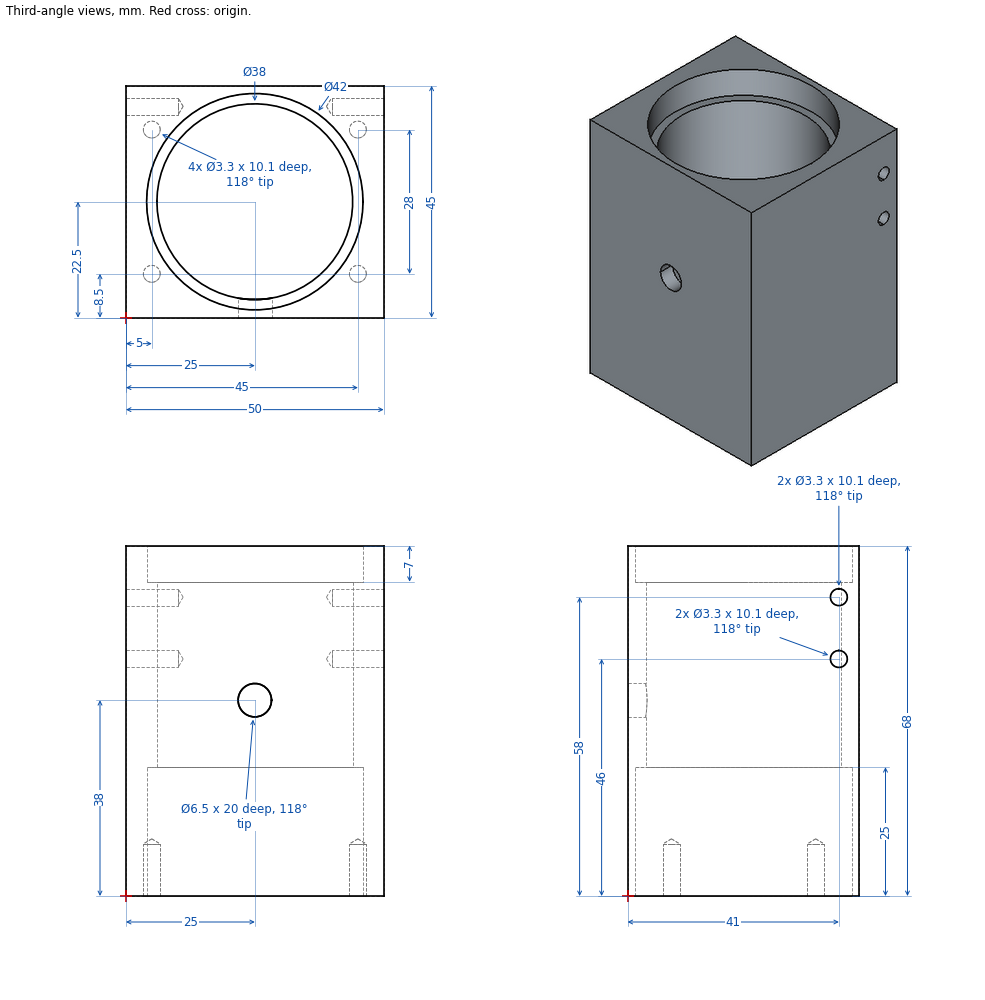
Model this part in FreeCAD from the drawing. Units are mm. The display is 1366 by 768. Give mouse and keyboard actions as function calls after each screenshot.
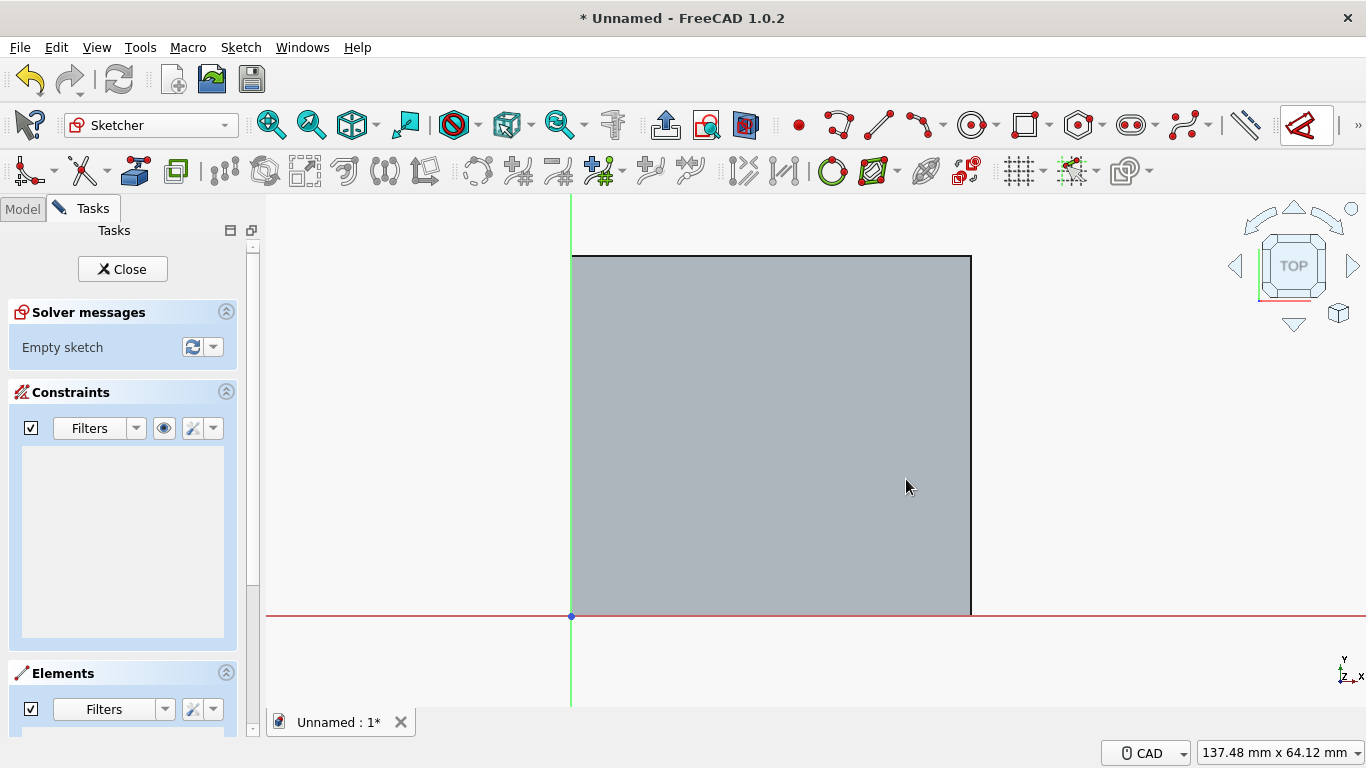
click(972, 126)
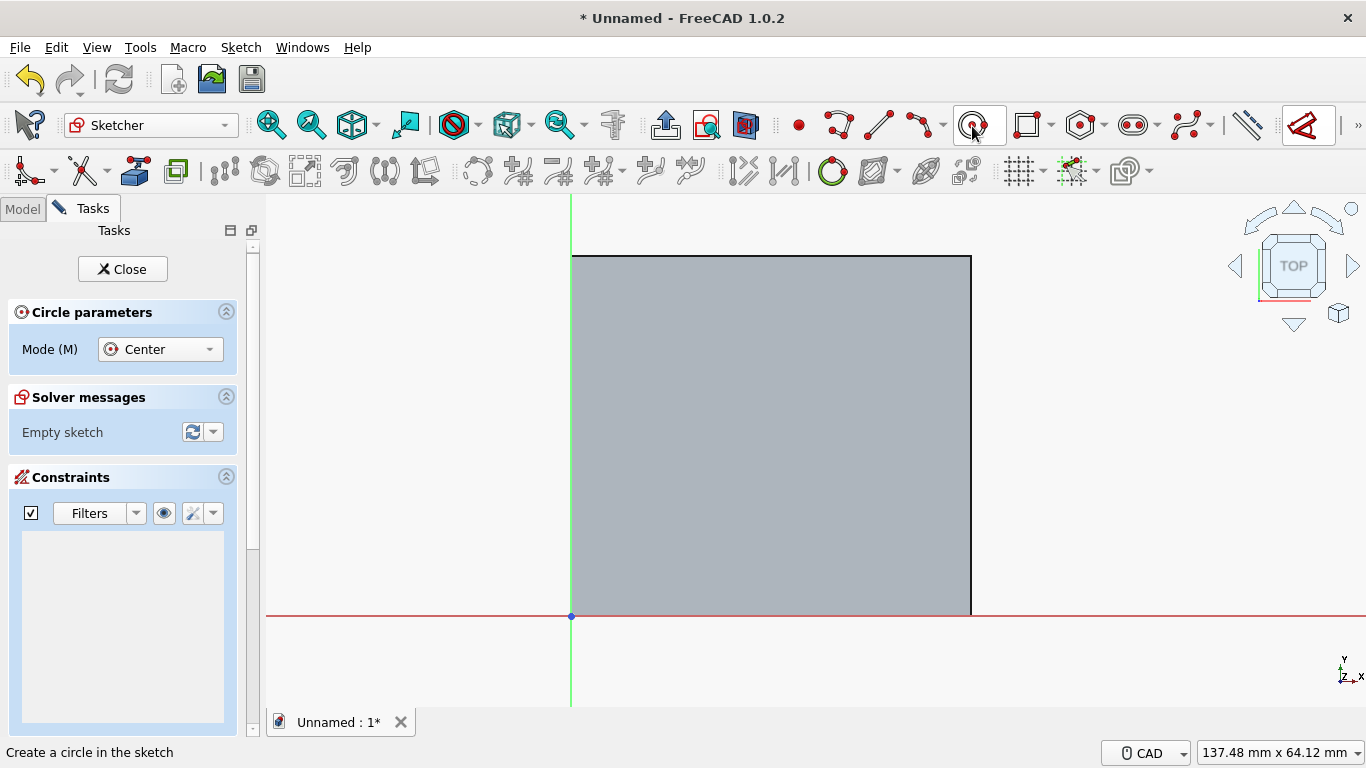
click(771, 436)
move(879, 329)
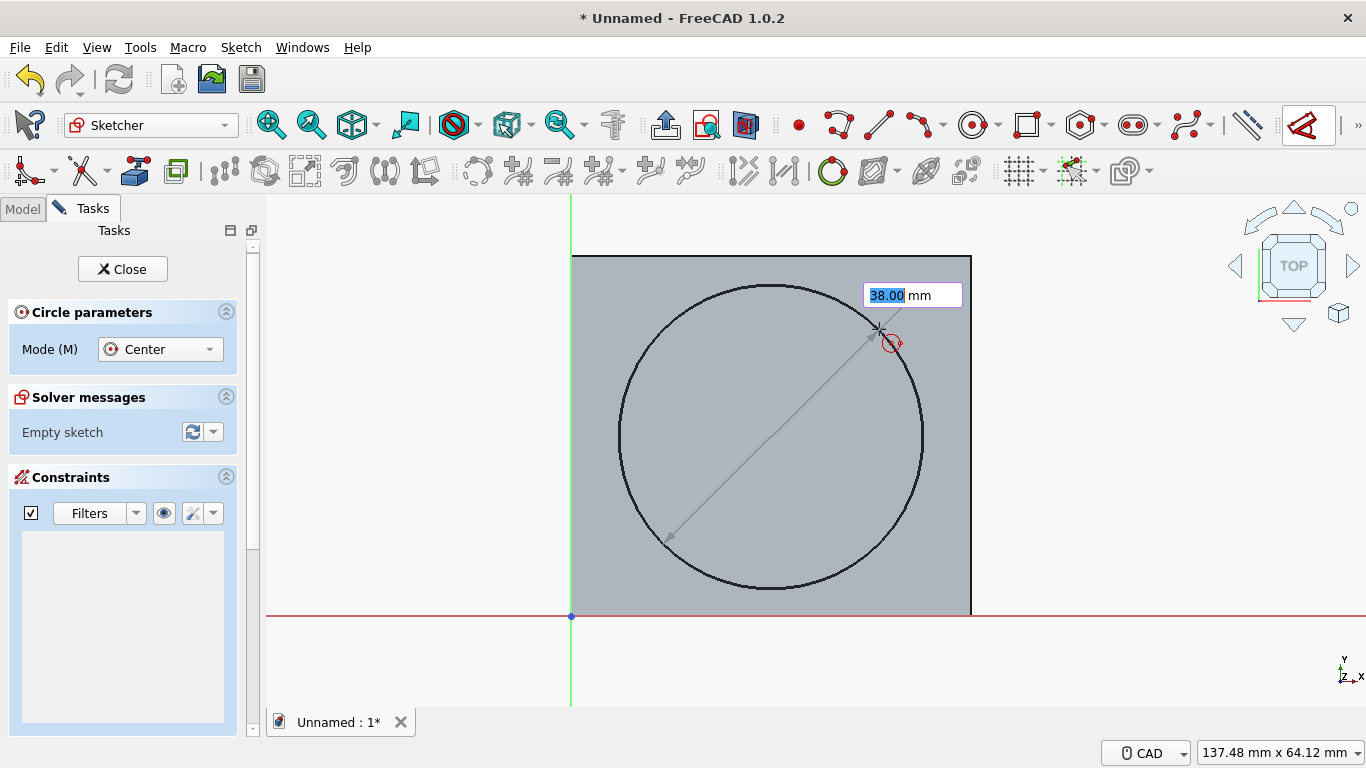
text(38)
key(Return)
key(Escape)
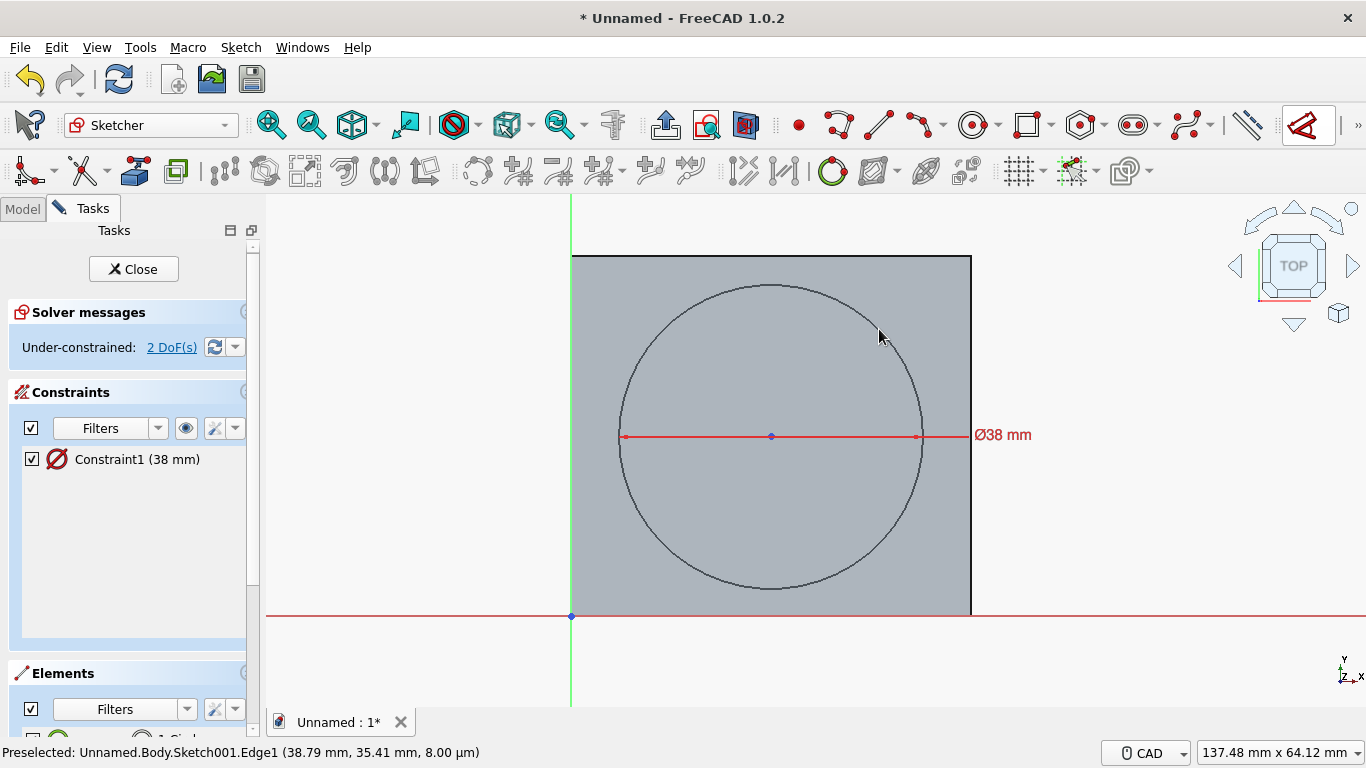
click(1302, 126)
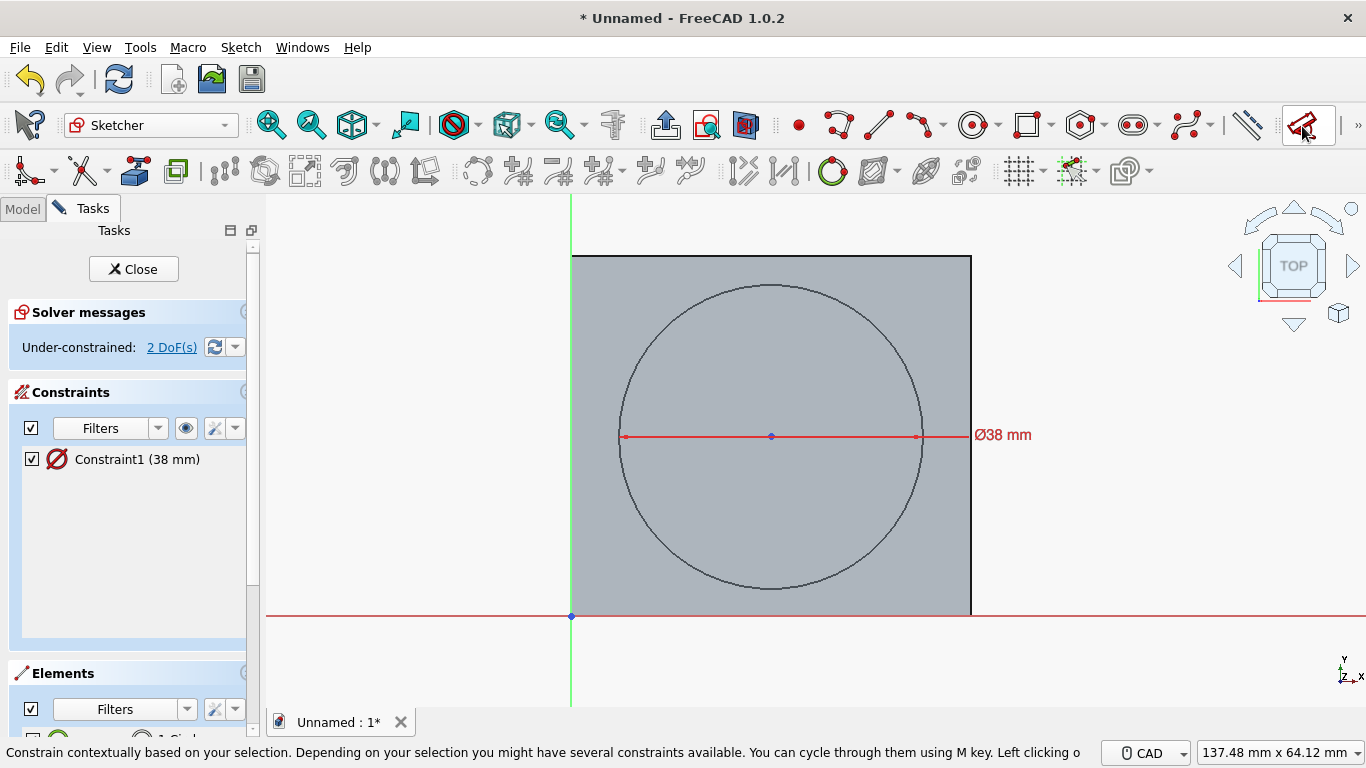
click(771, 437)
click(671, 650)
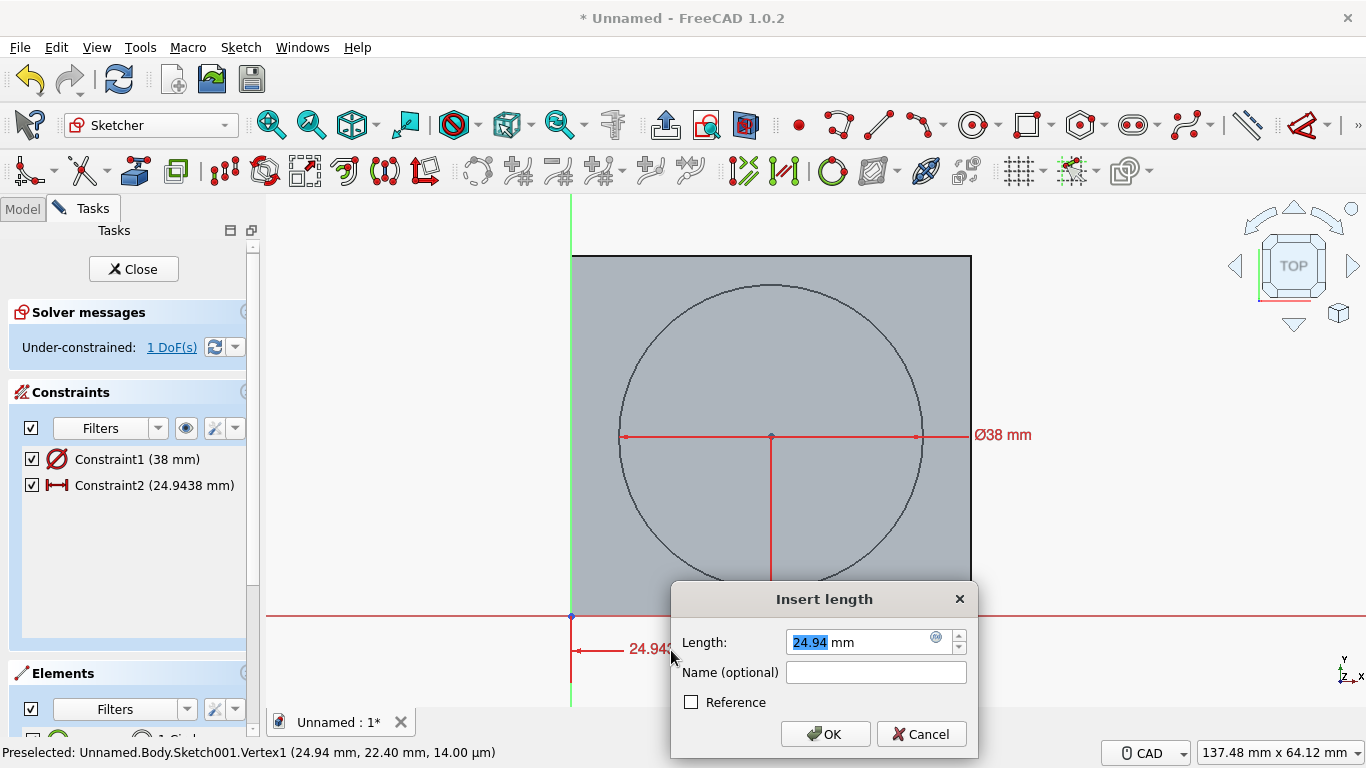
text(25)
key(Return)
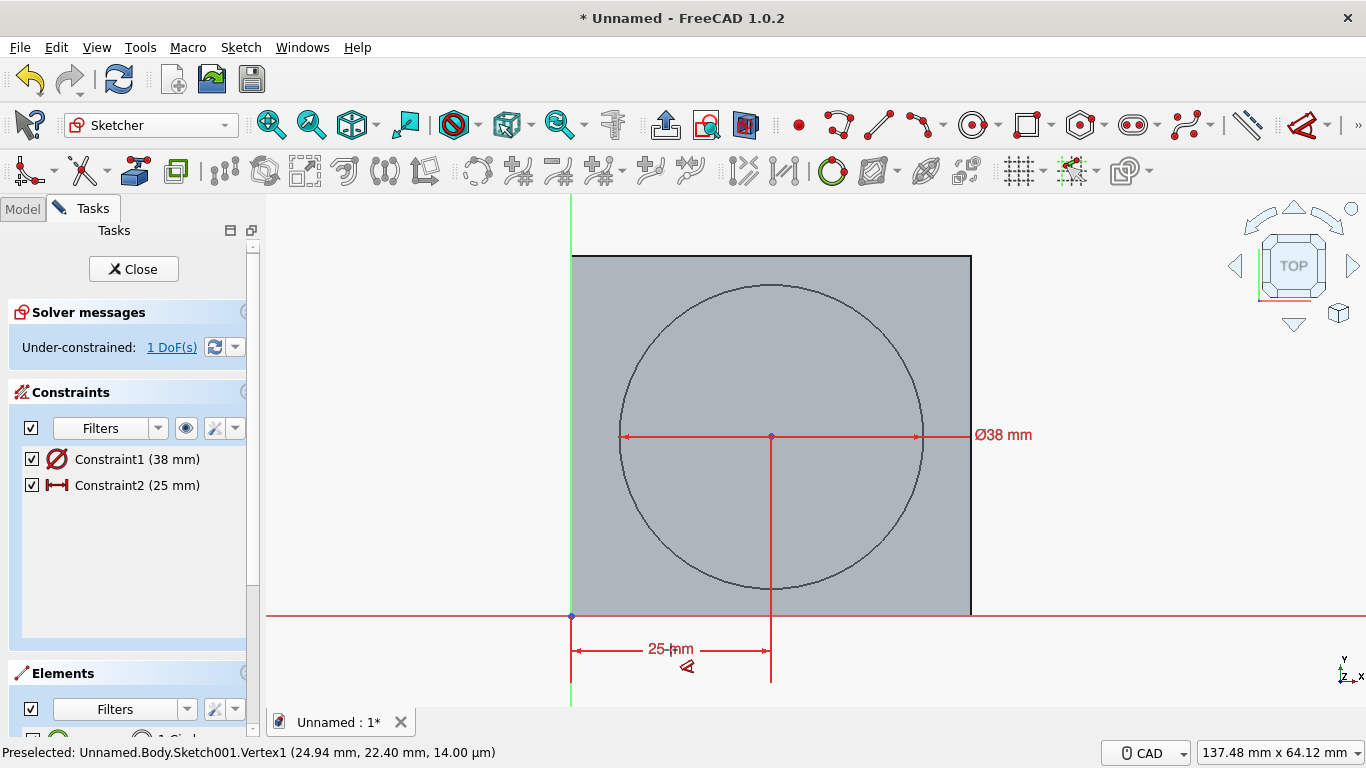
click(771, 437)
click(537, 527)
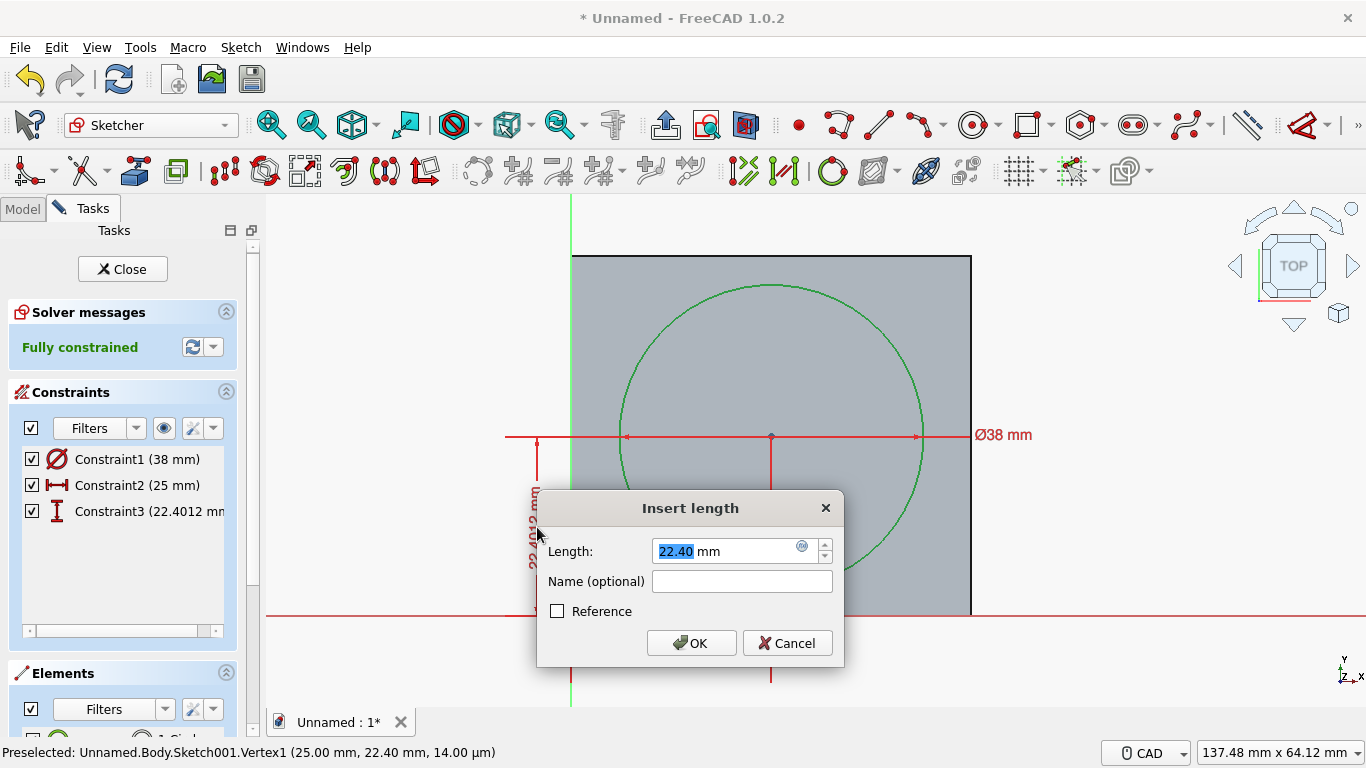
text(22.5)
key(Return)
key(Escape)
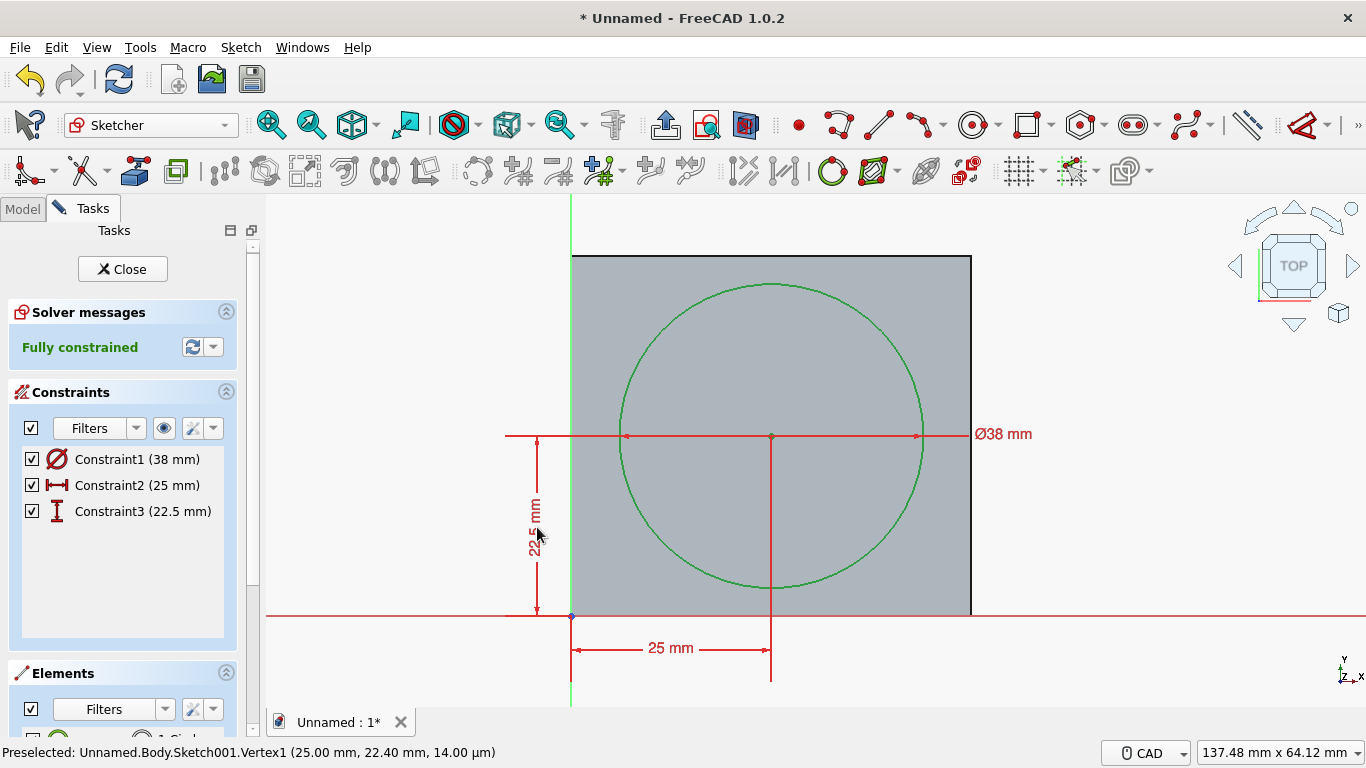
click(123, 269)